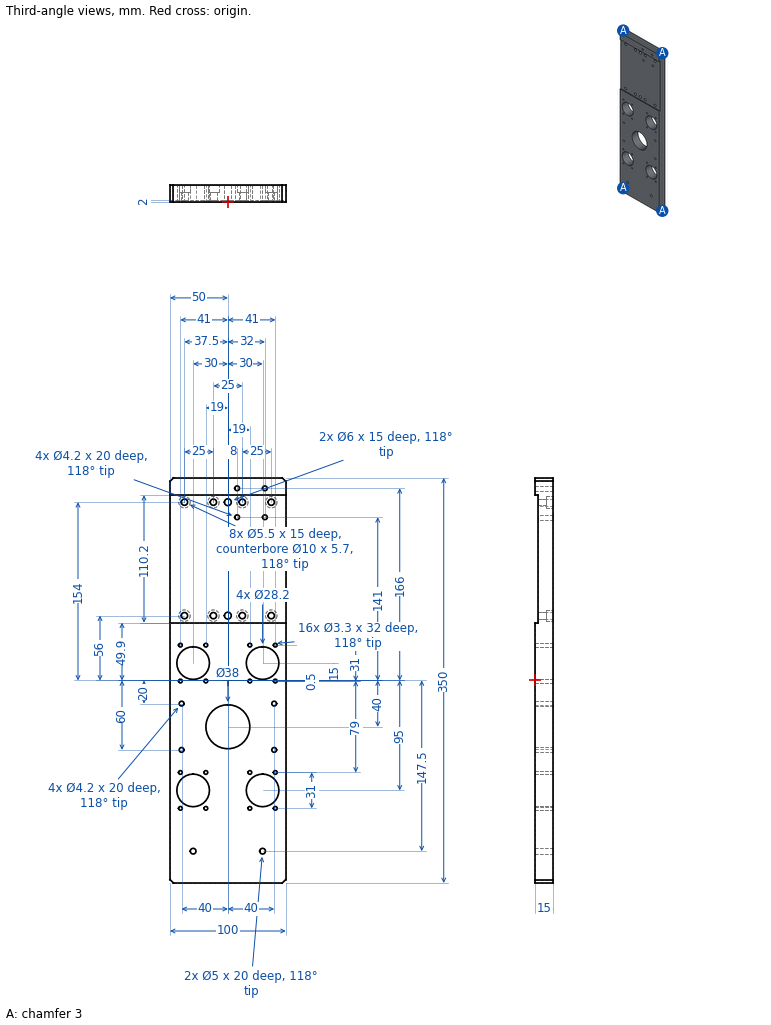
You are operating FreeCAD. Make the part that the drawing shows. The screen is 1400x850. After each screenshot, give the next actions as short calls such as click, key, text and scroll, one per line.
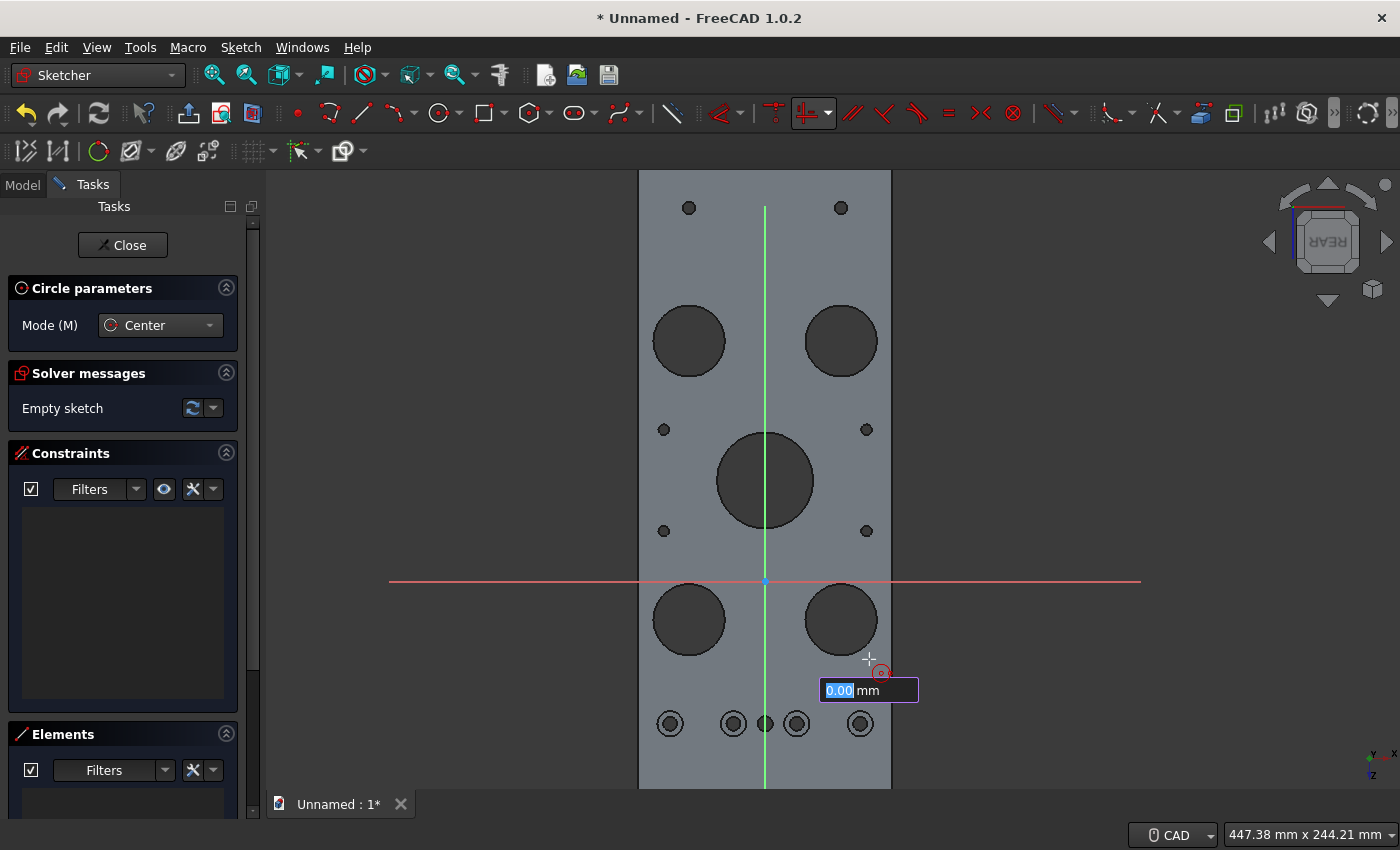
scroll(872, 656, up, 7)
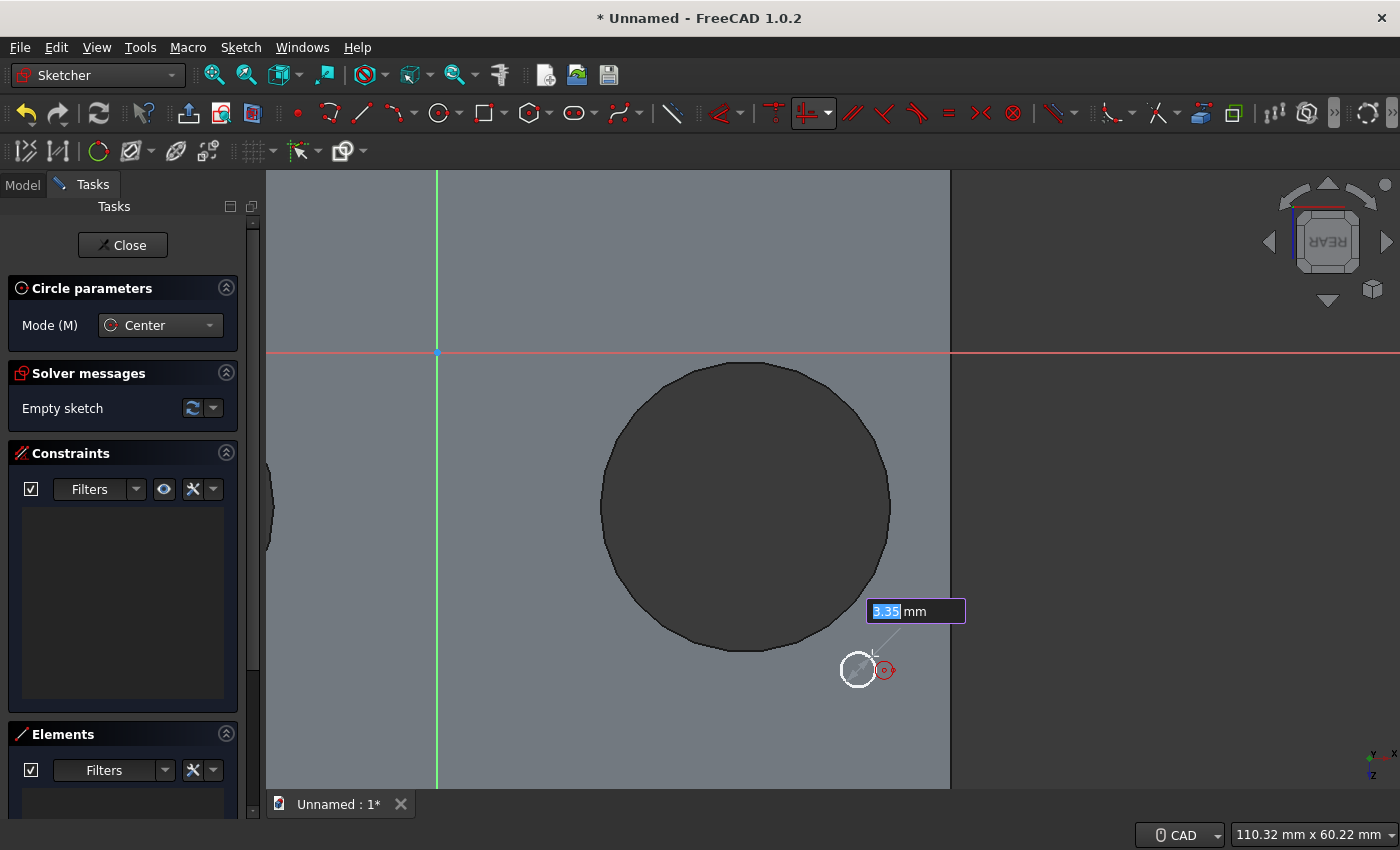
click(871, 654)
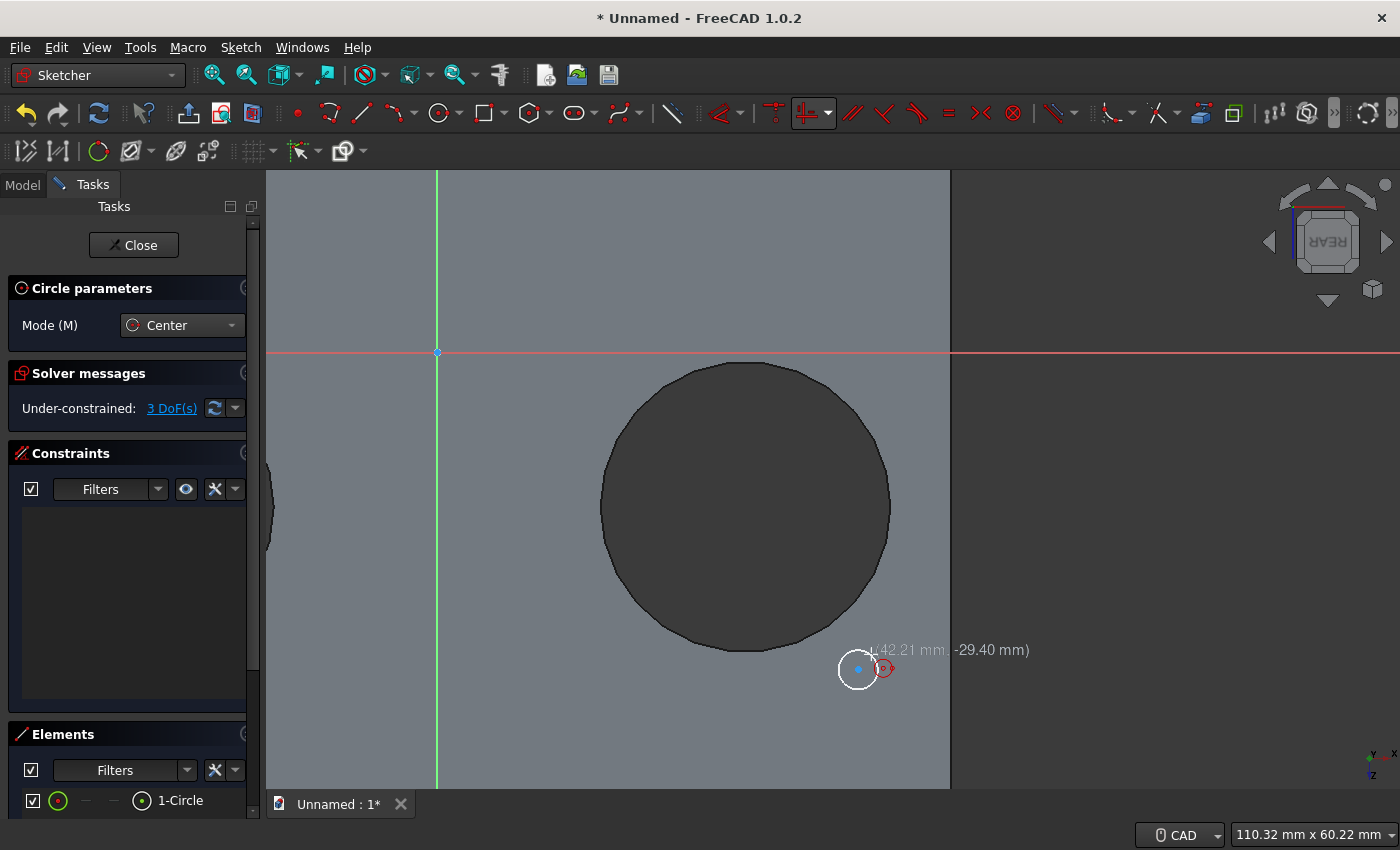
scroll(632, 666, up, 2)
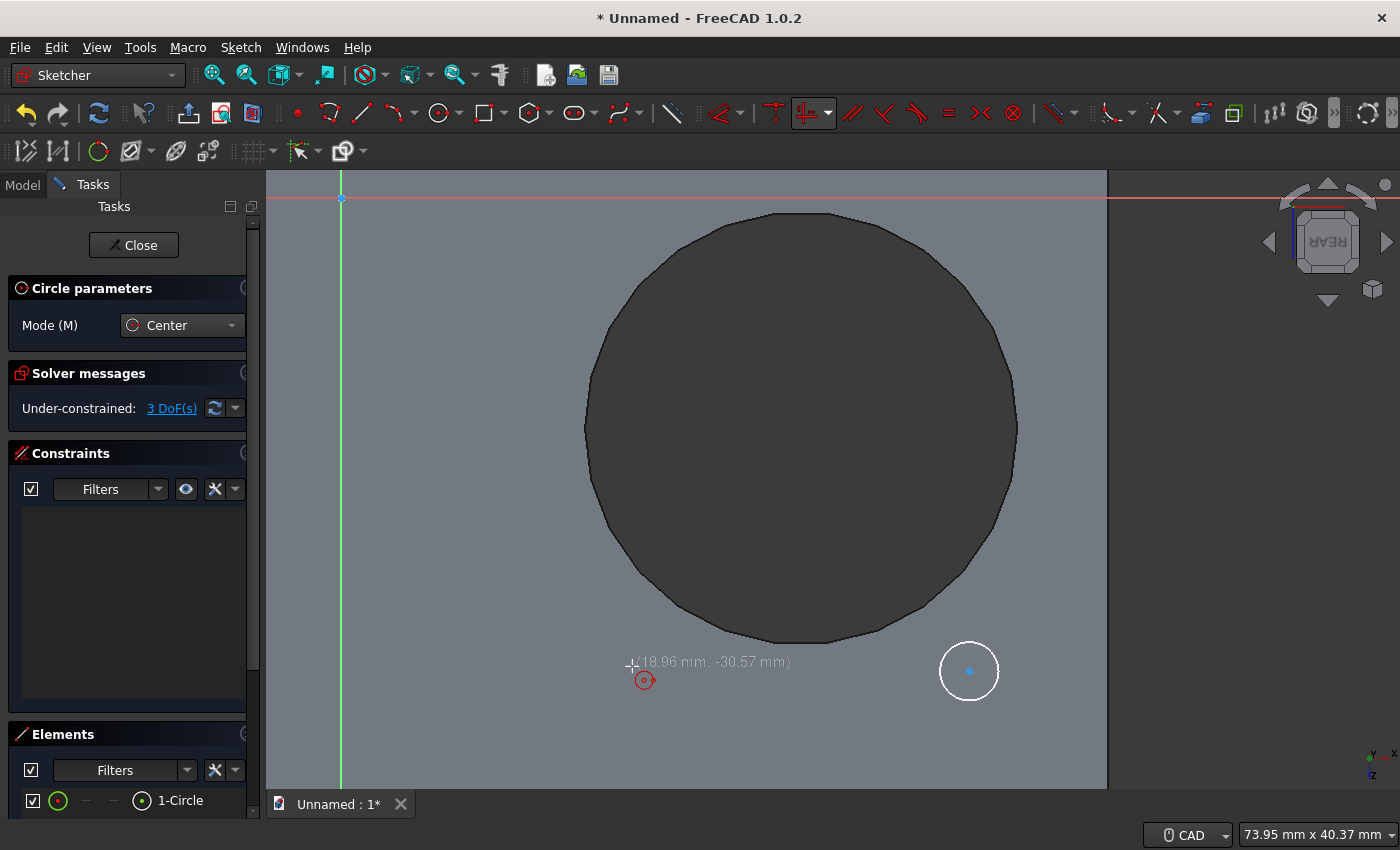
scroll(848, 657, down, 9)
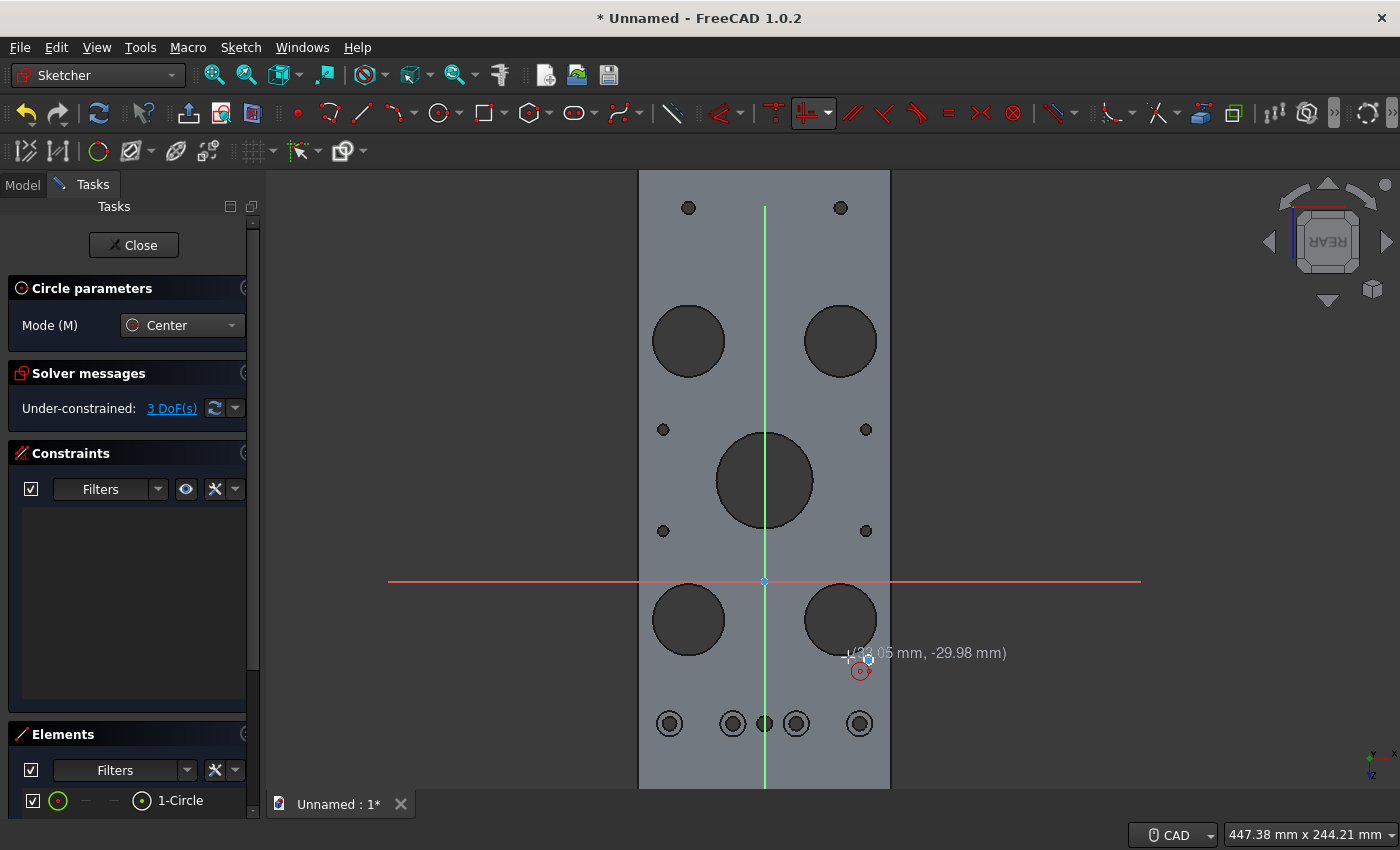
click(813, 659)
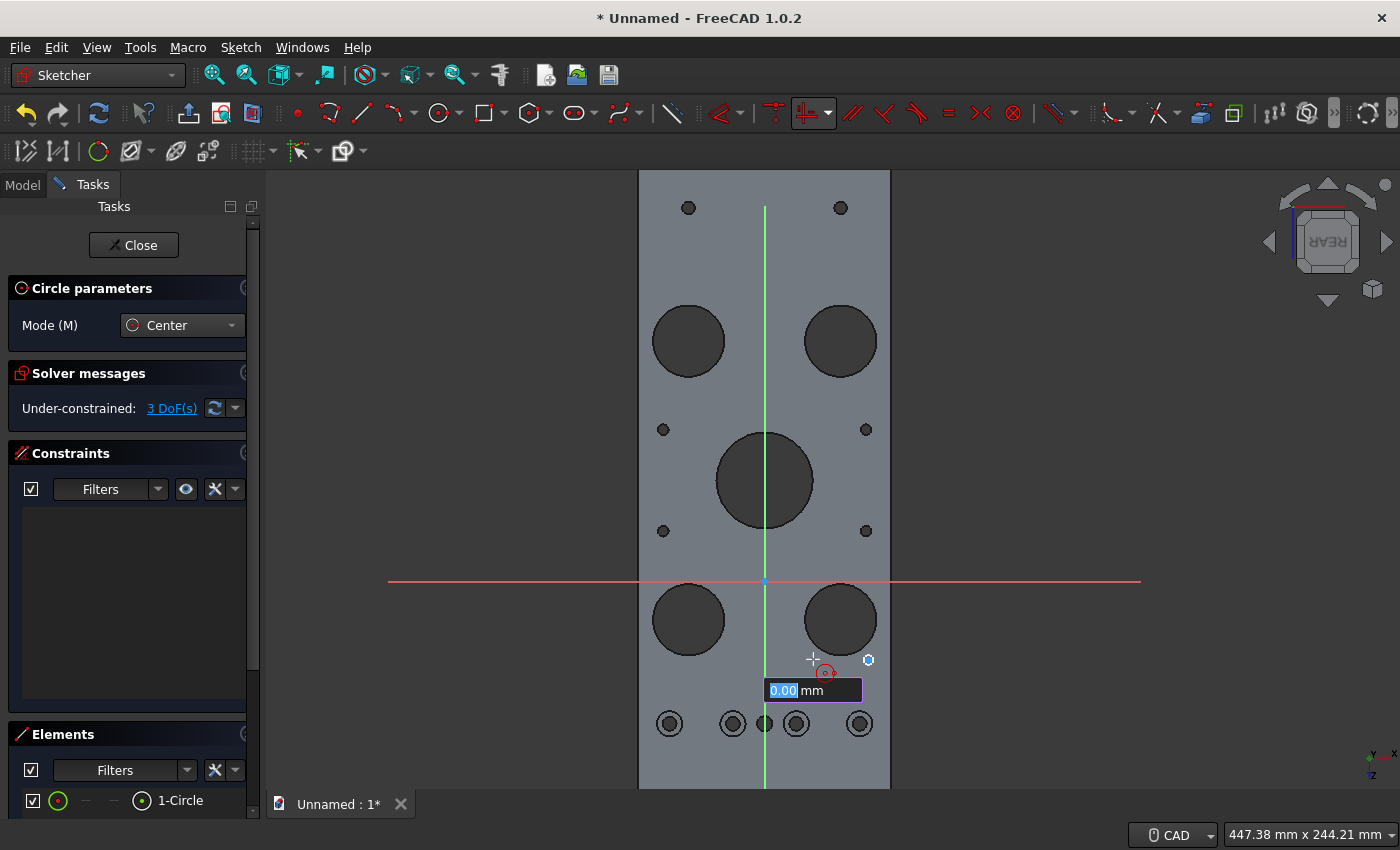
scroll(816, 656, up, 7)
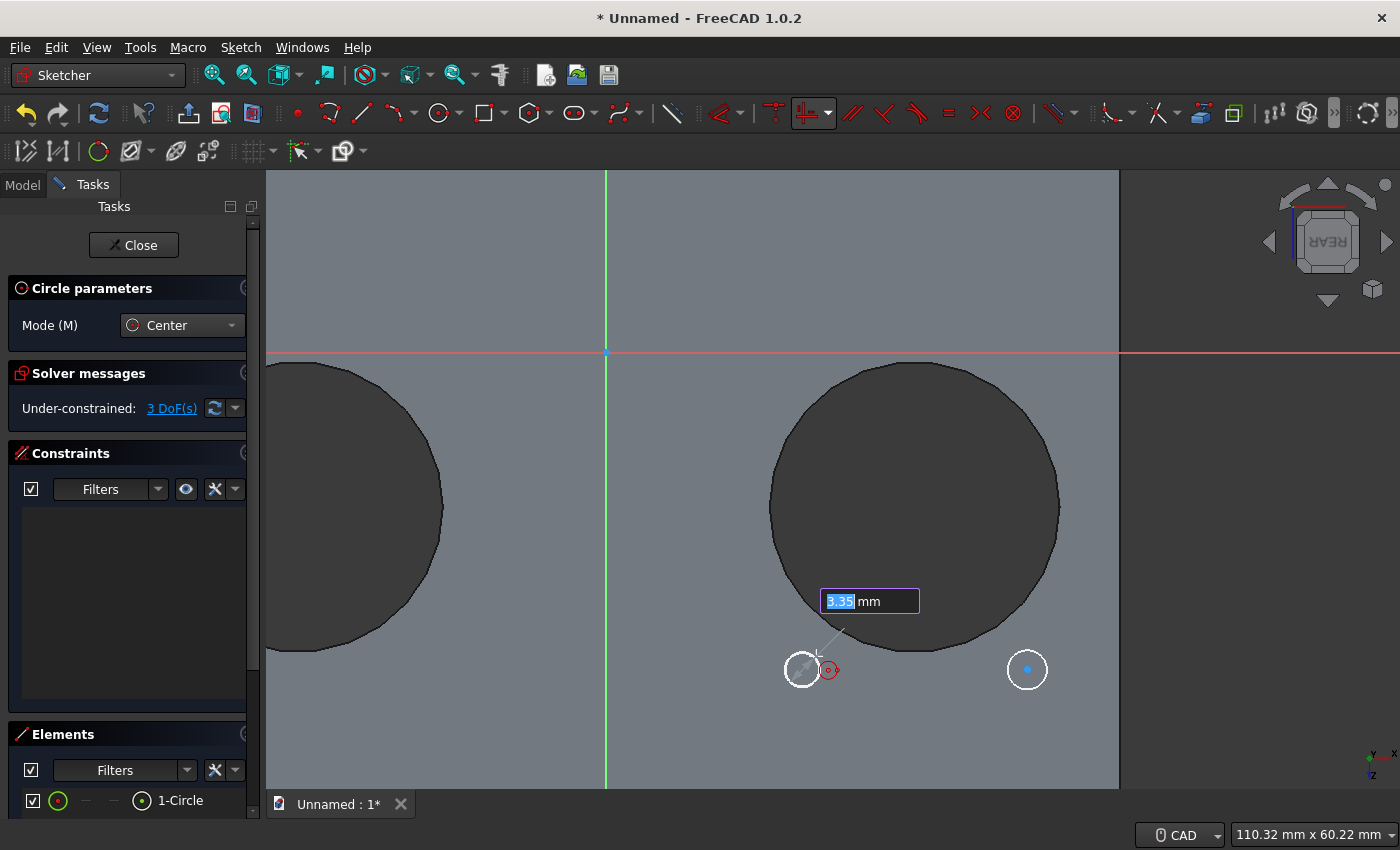
click(814, 654)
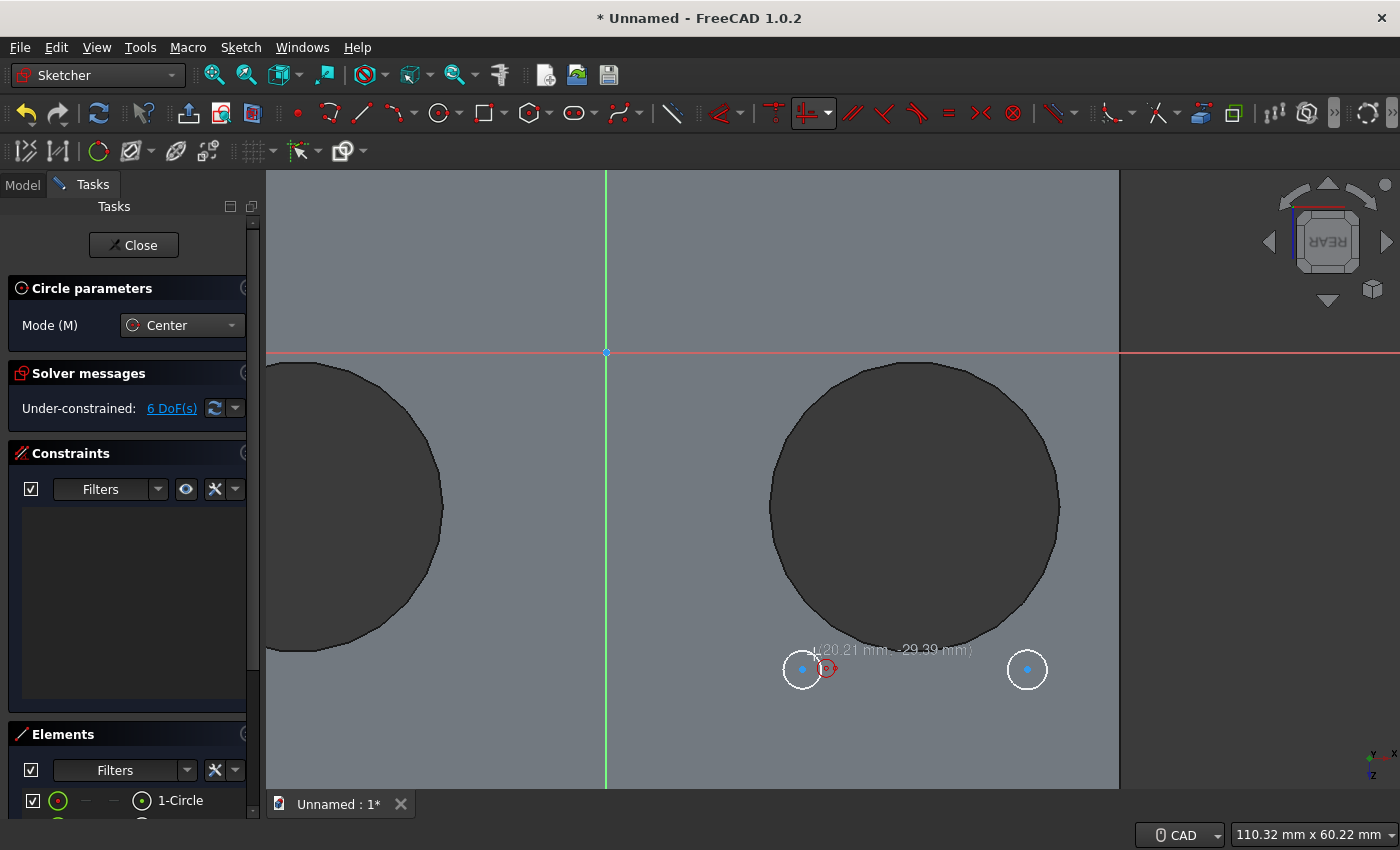
scroll(1028, 348, up, 6)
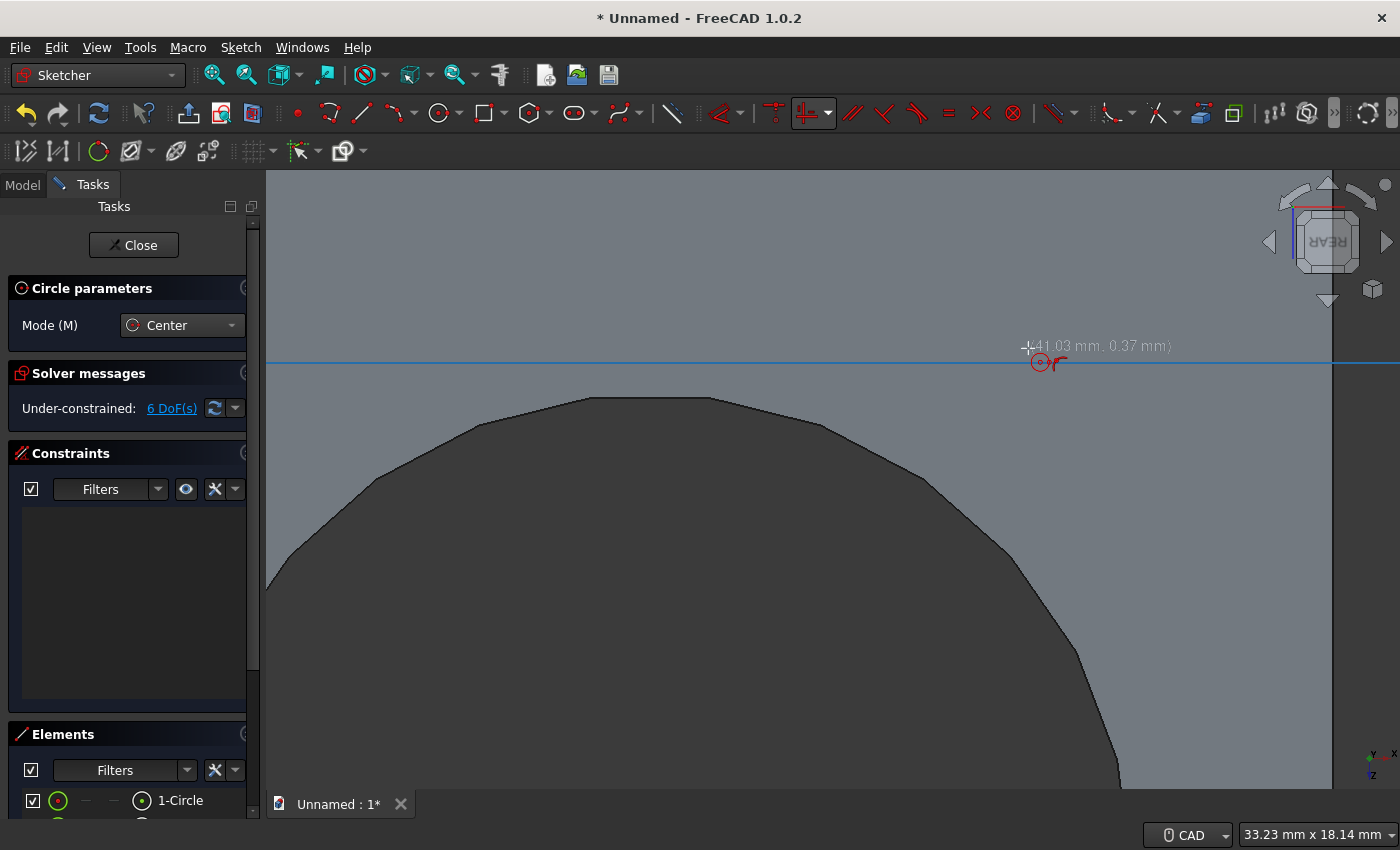
click(1025, 346)